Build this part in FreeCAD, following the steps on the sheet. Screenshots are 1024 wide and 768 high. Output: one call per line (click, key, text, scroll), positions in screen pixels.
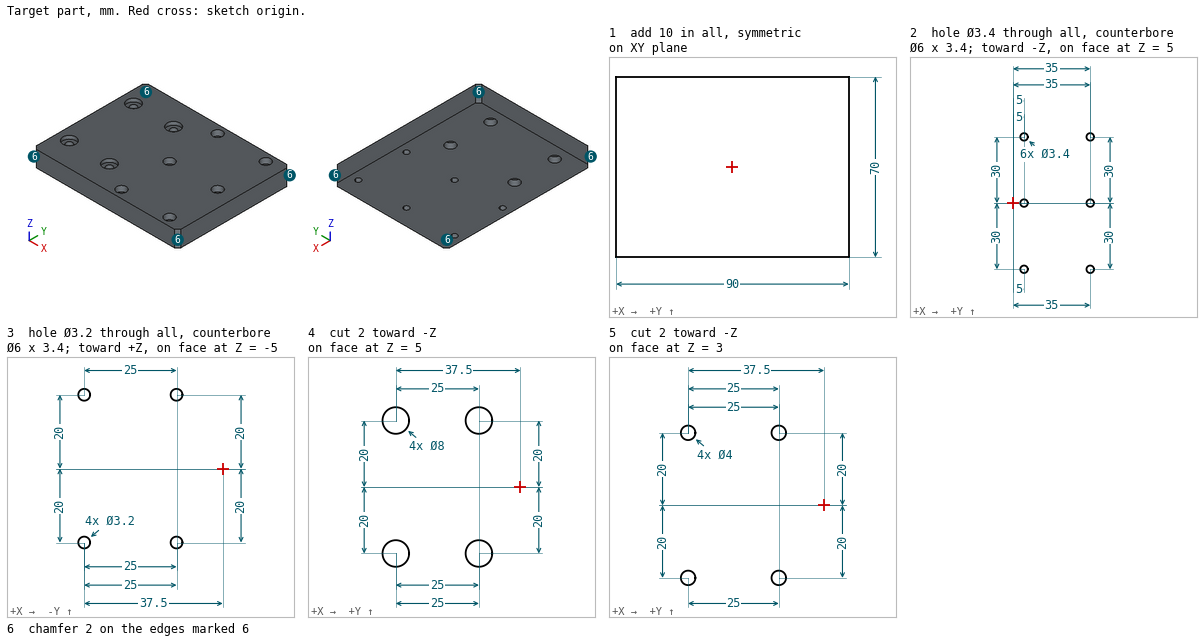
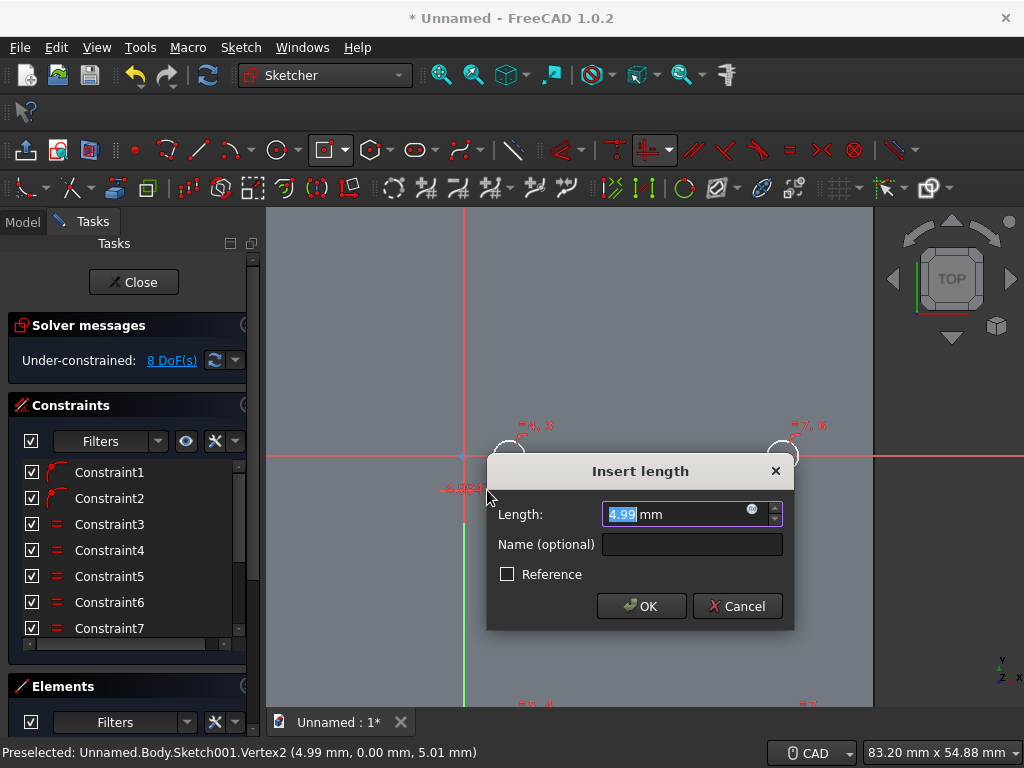
text(5)
key(Return)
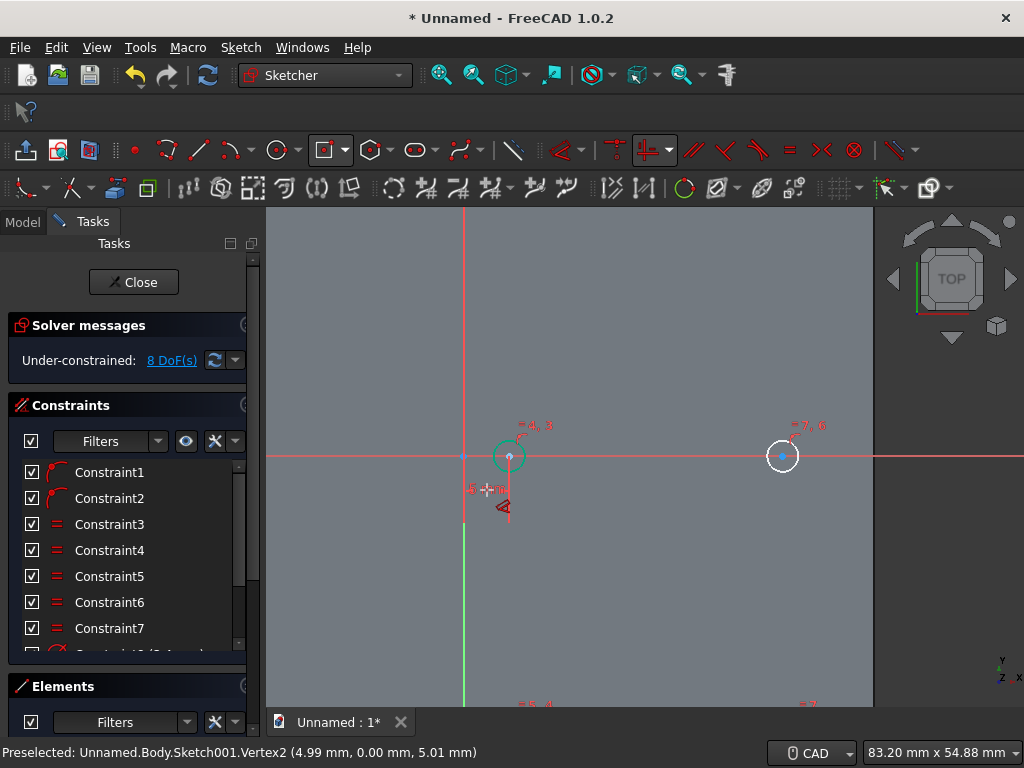
scroll(510, 458, down, 3)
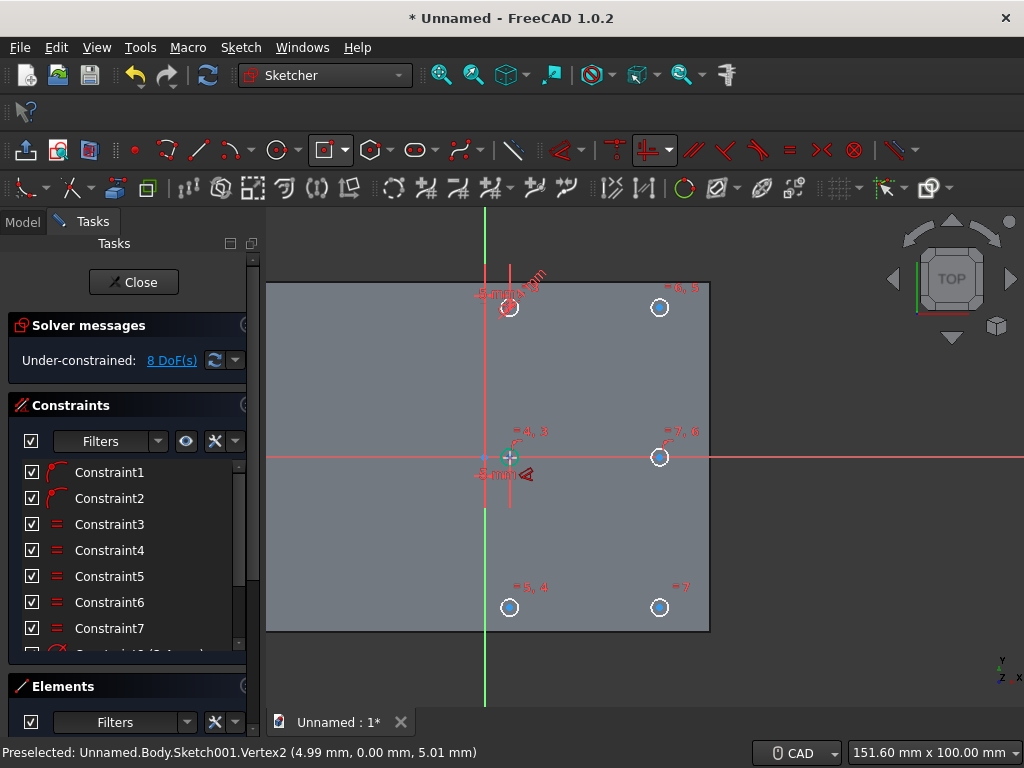
scroll(510, 608, up, 3)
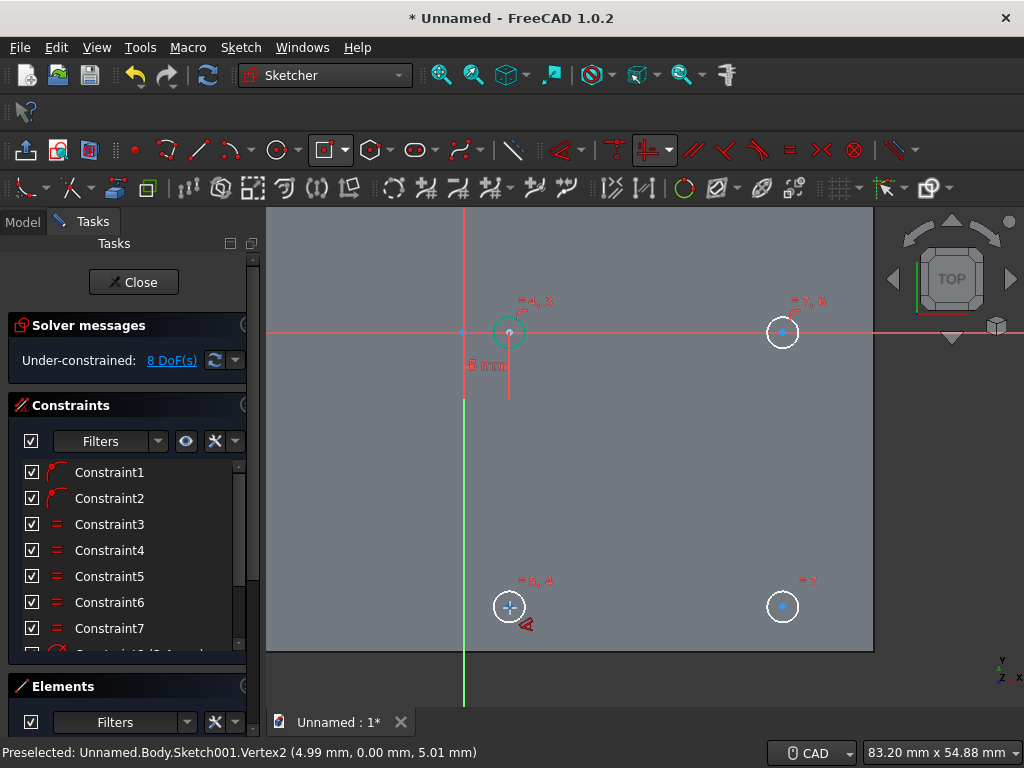
click(509, 607)
click(487, 641)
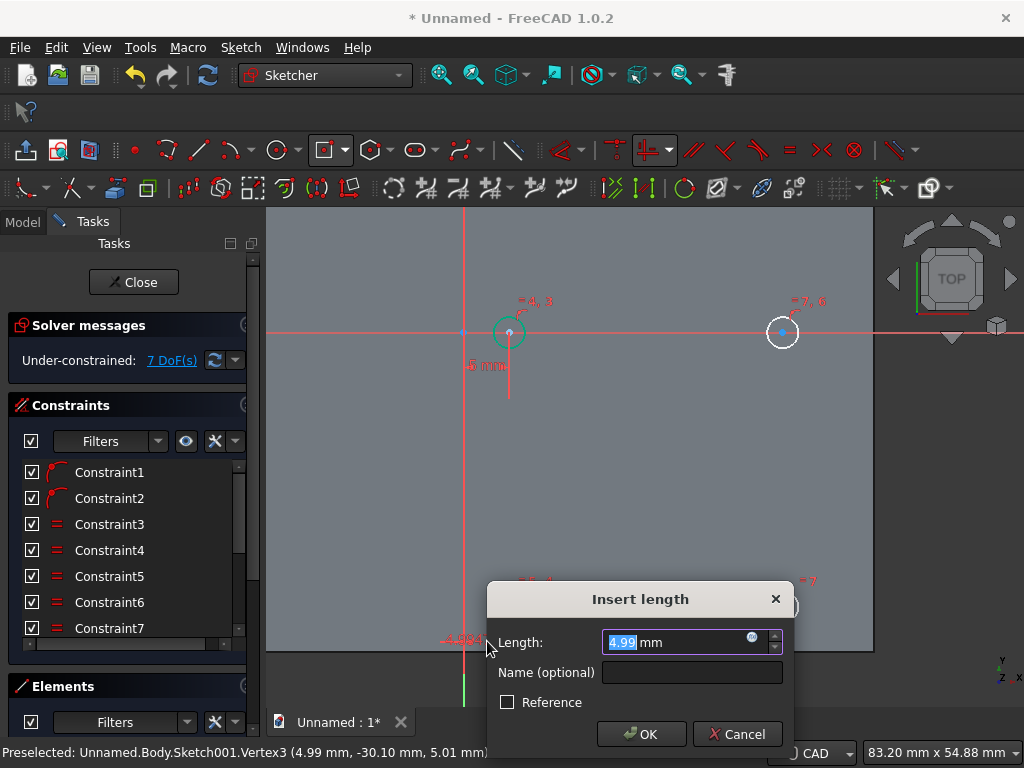
text(5)
key(Return)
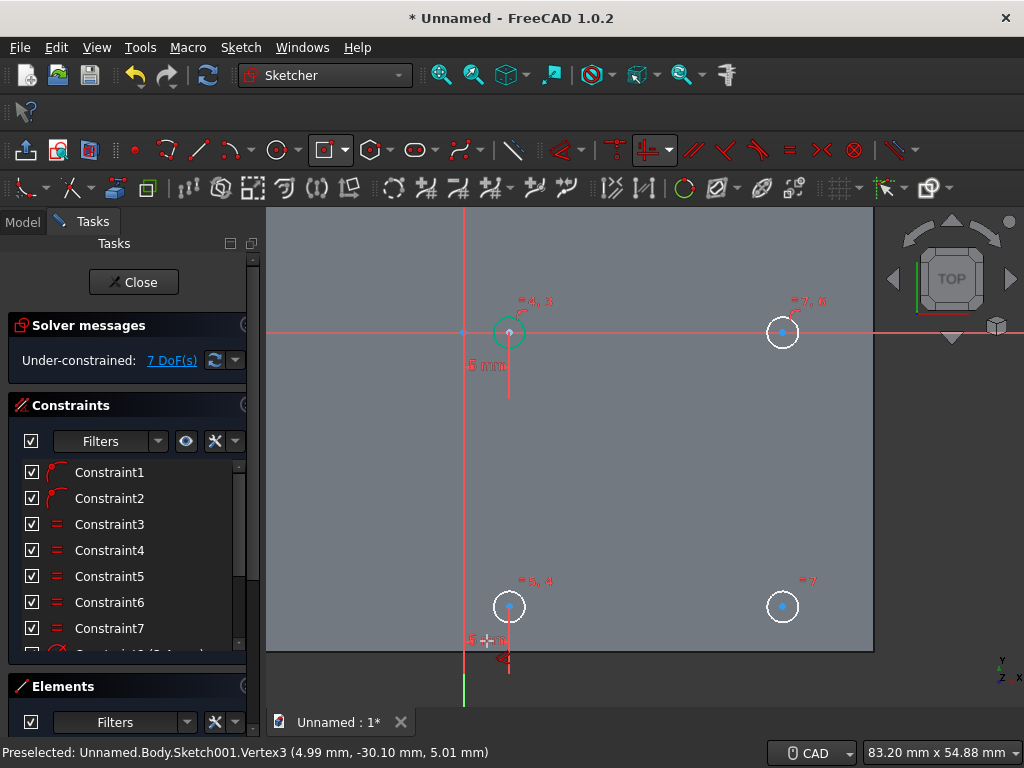
scroll(510, 608, down, 3)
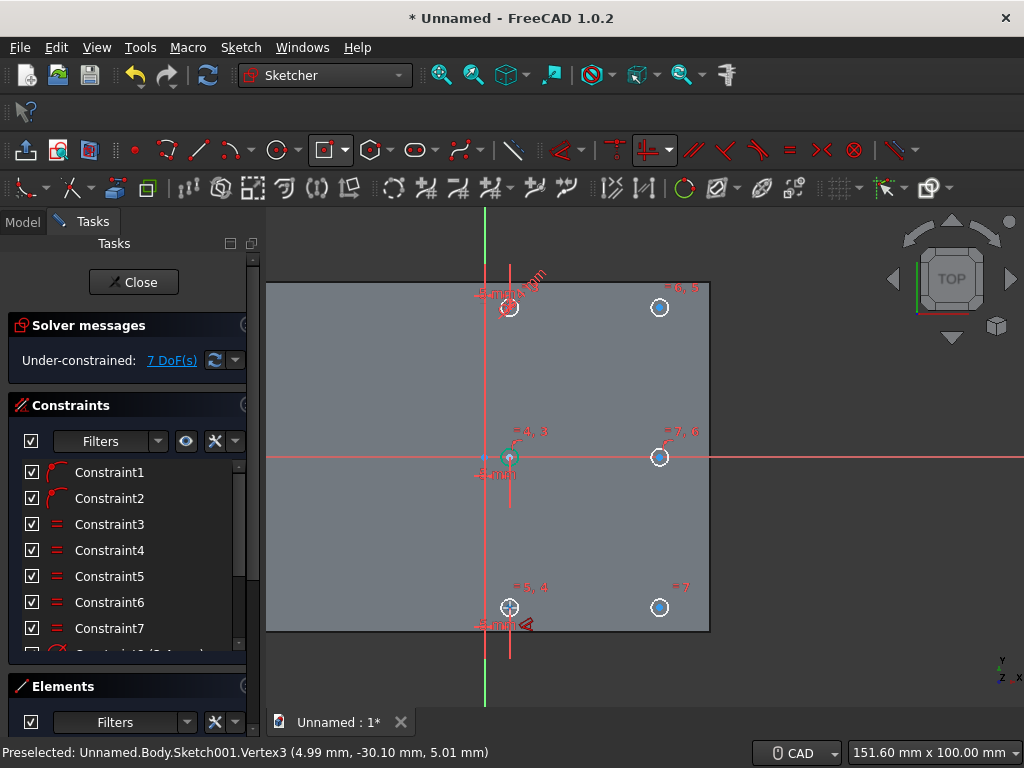
click(510, 308)
click(451, 383)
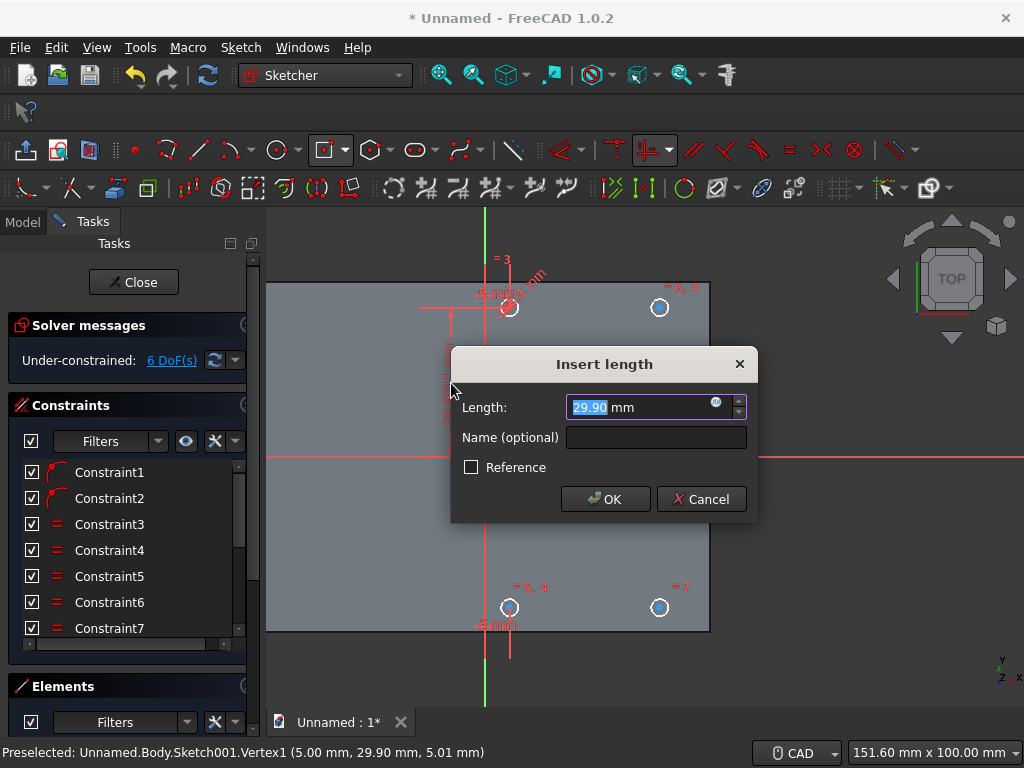
text(30)
key(Return)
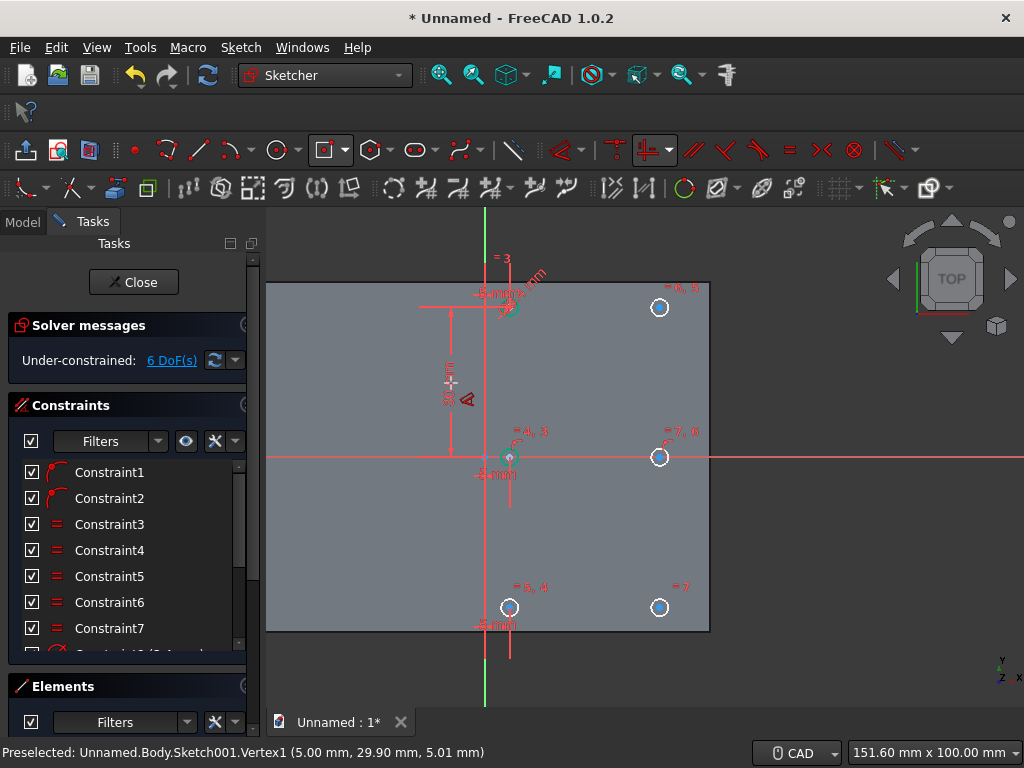
click(510, 608)
click(451, 533)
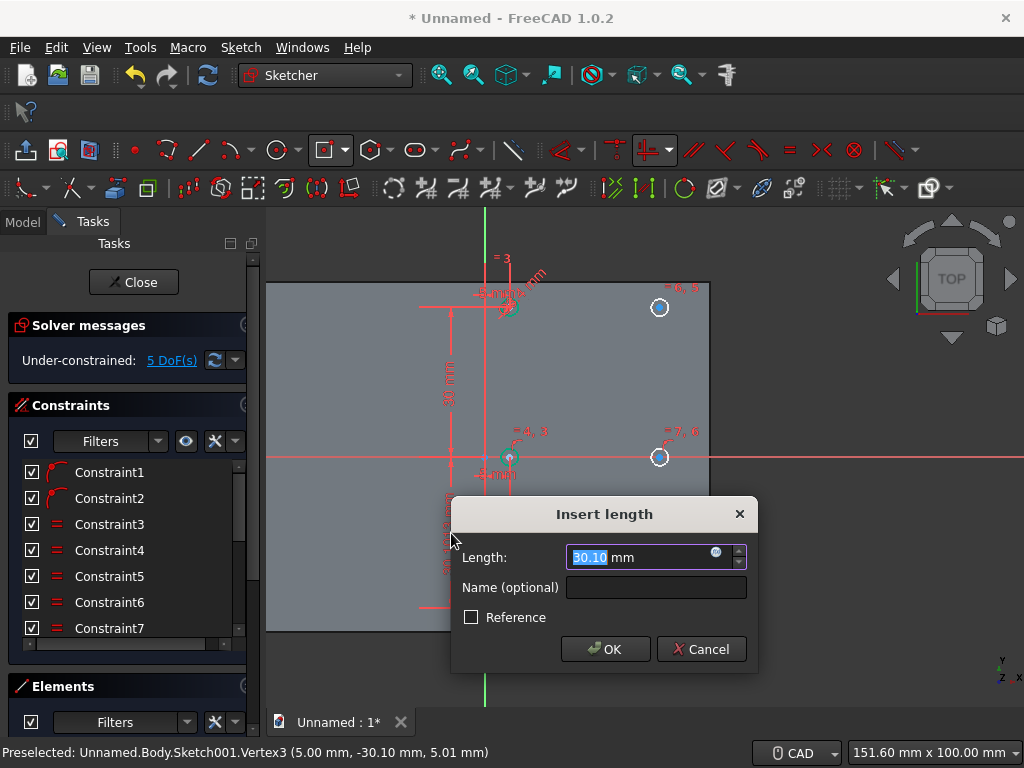
text(30)
key(Return)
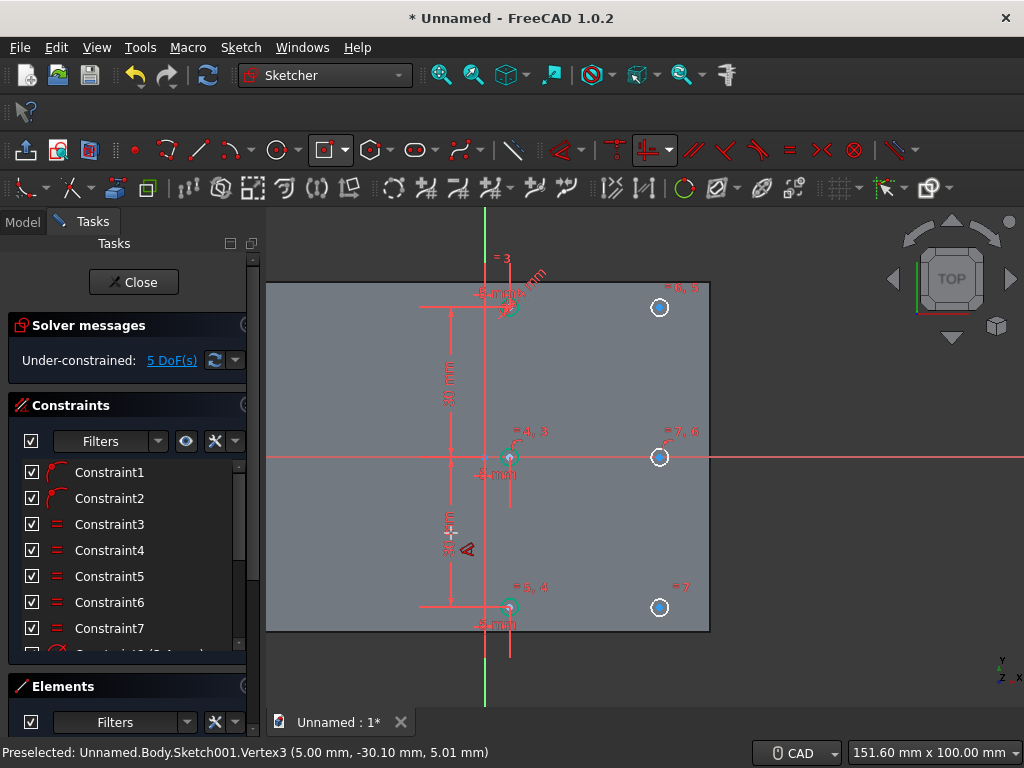
click(660, 308)
click(613, 274)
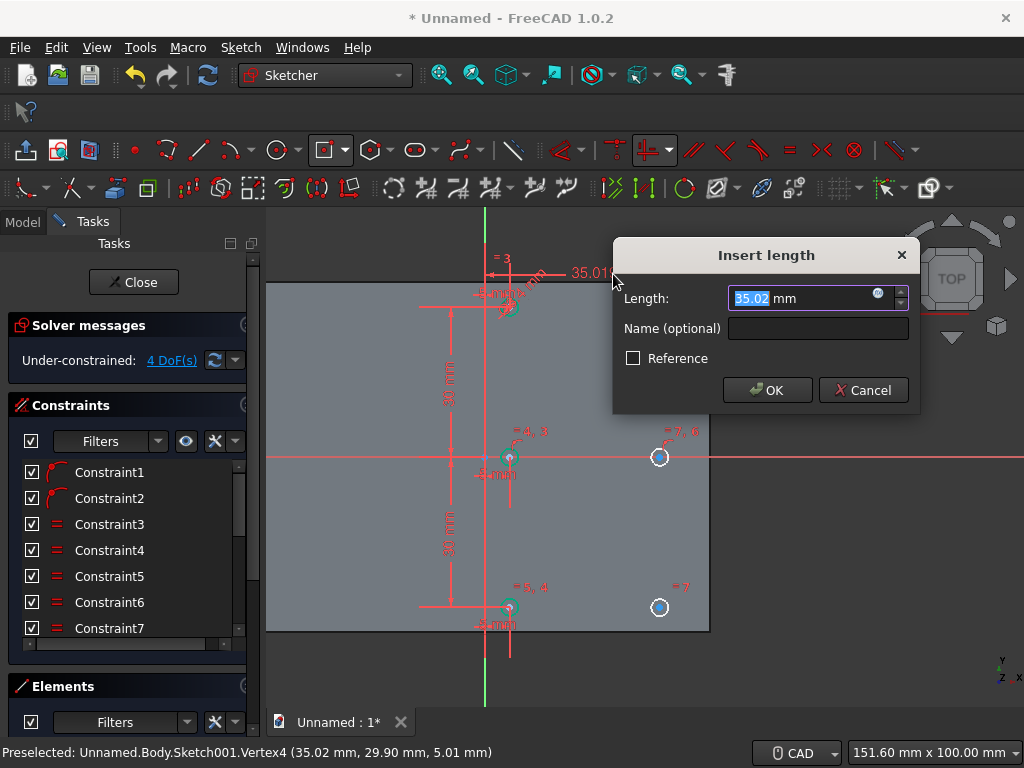
text(35)
key(Return)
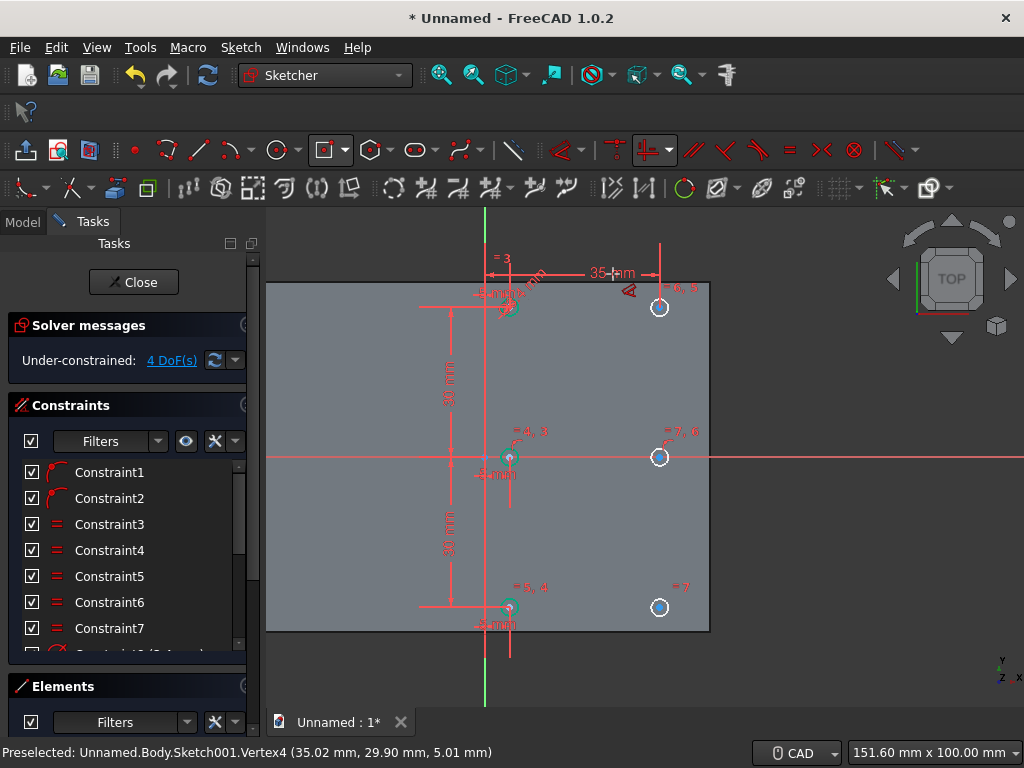
click(660, 308)
click(451, 348)